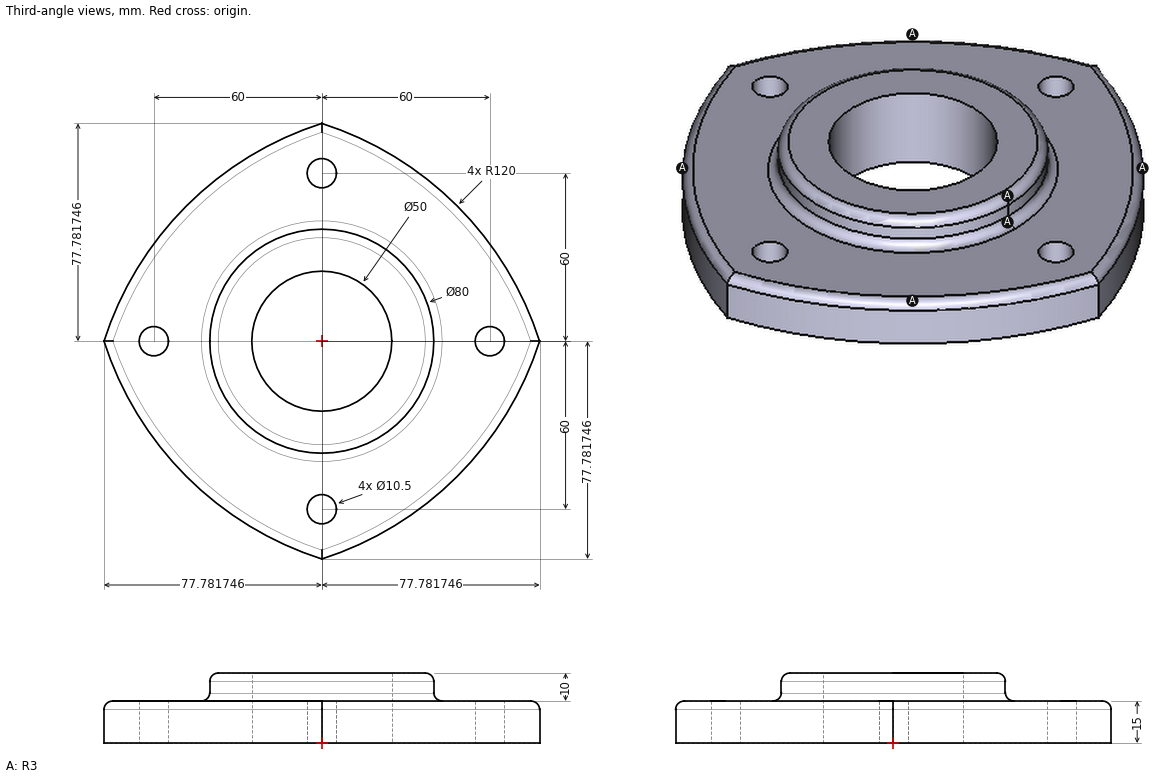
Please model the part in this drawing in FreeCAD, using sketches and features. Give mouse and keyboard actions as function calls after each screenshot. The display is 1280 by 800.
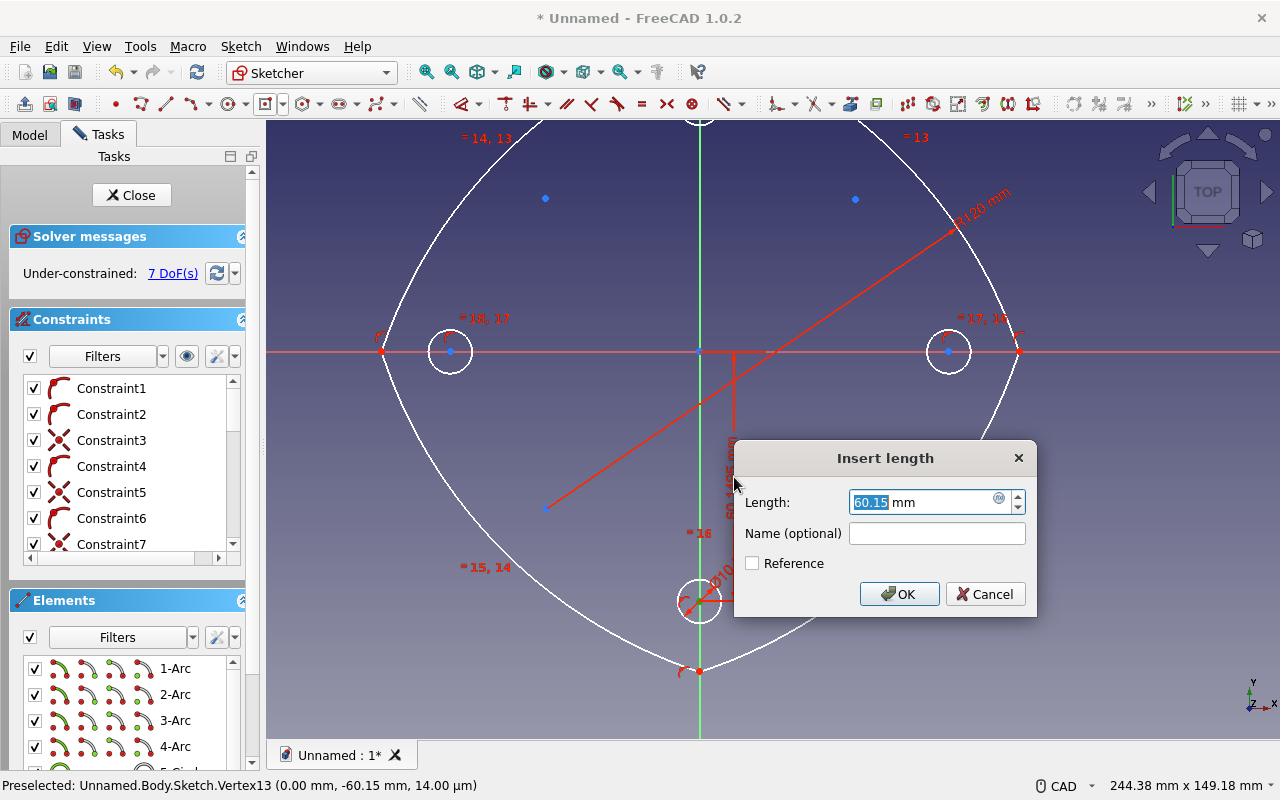
text(60)
key(Return)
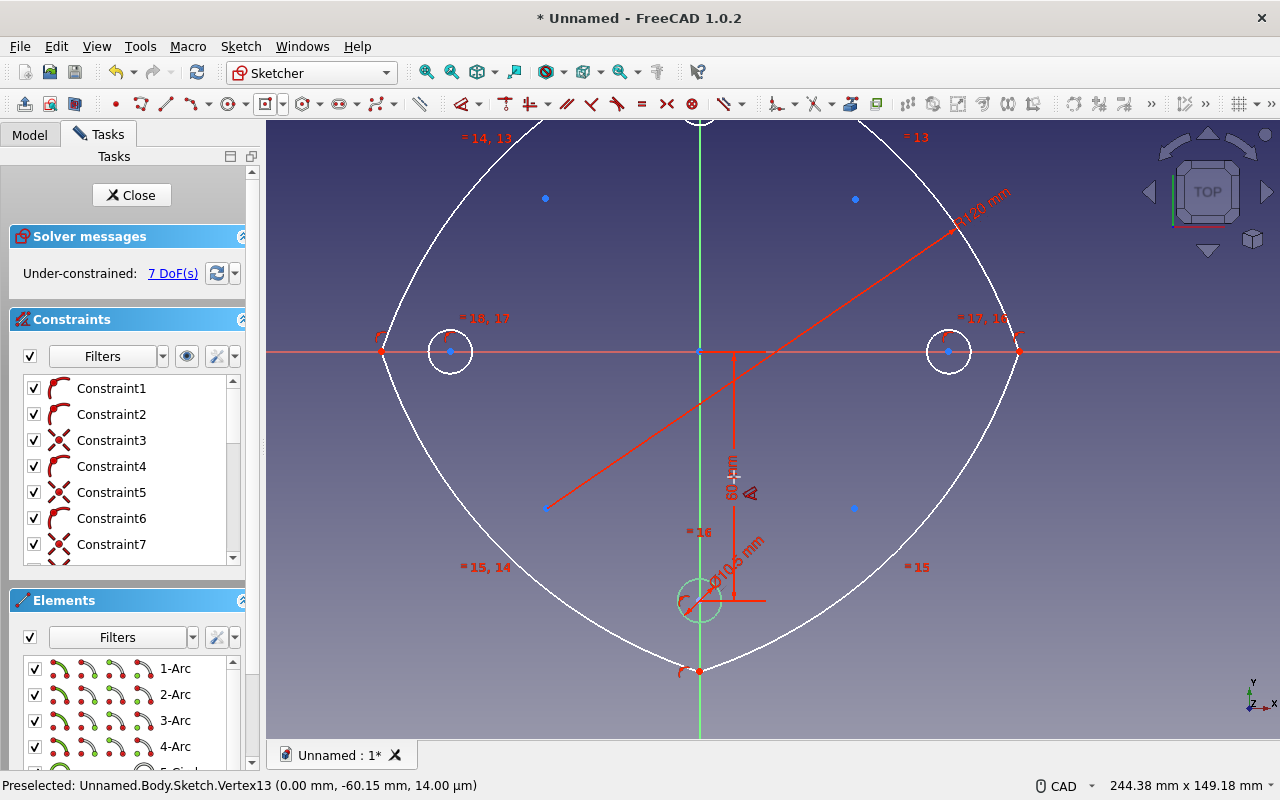
click(949, 352)
click(824, 386)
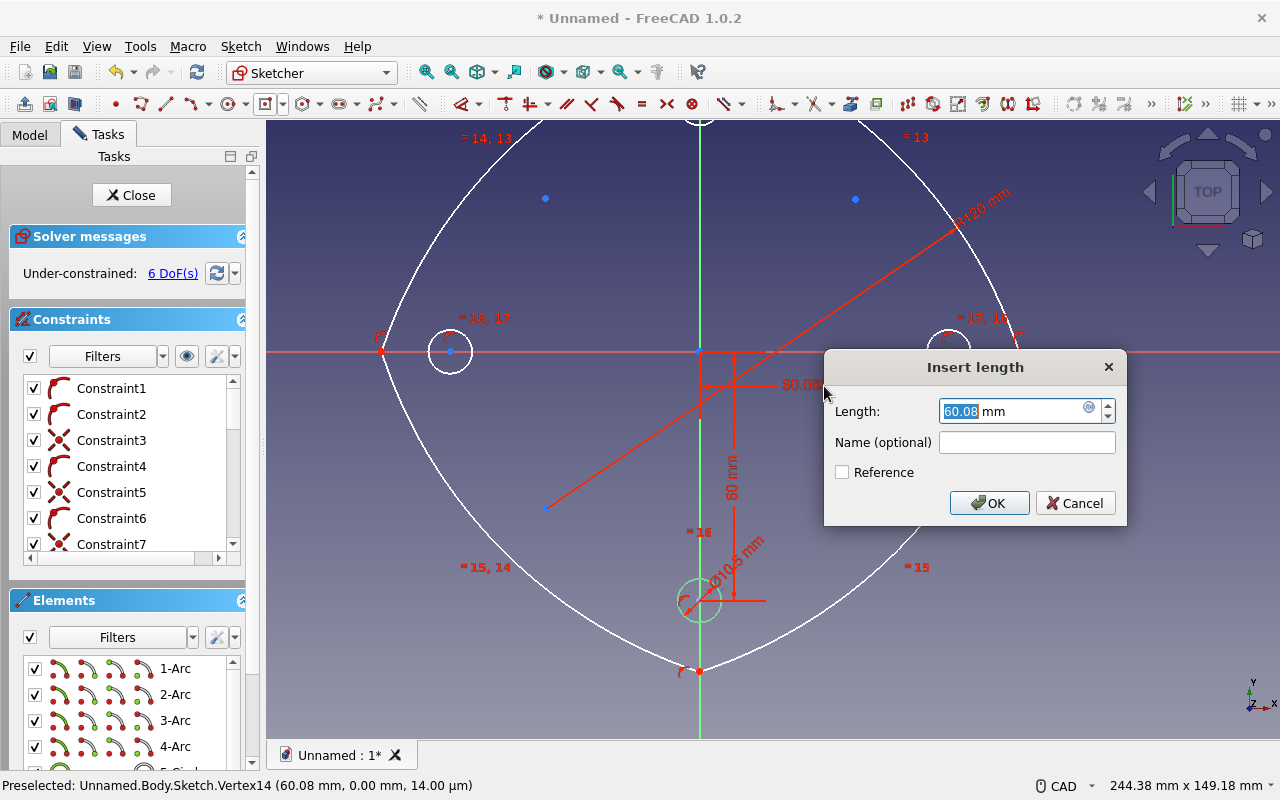
text(60)
key(Return)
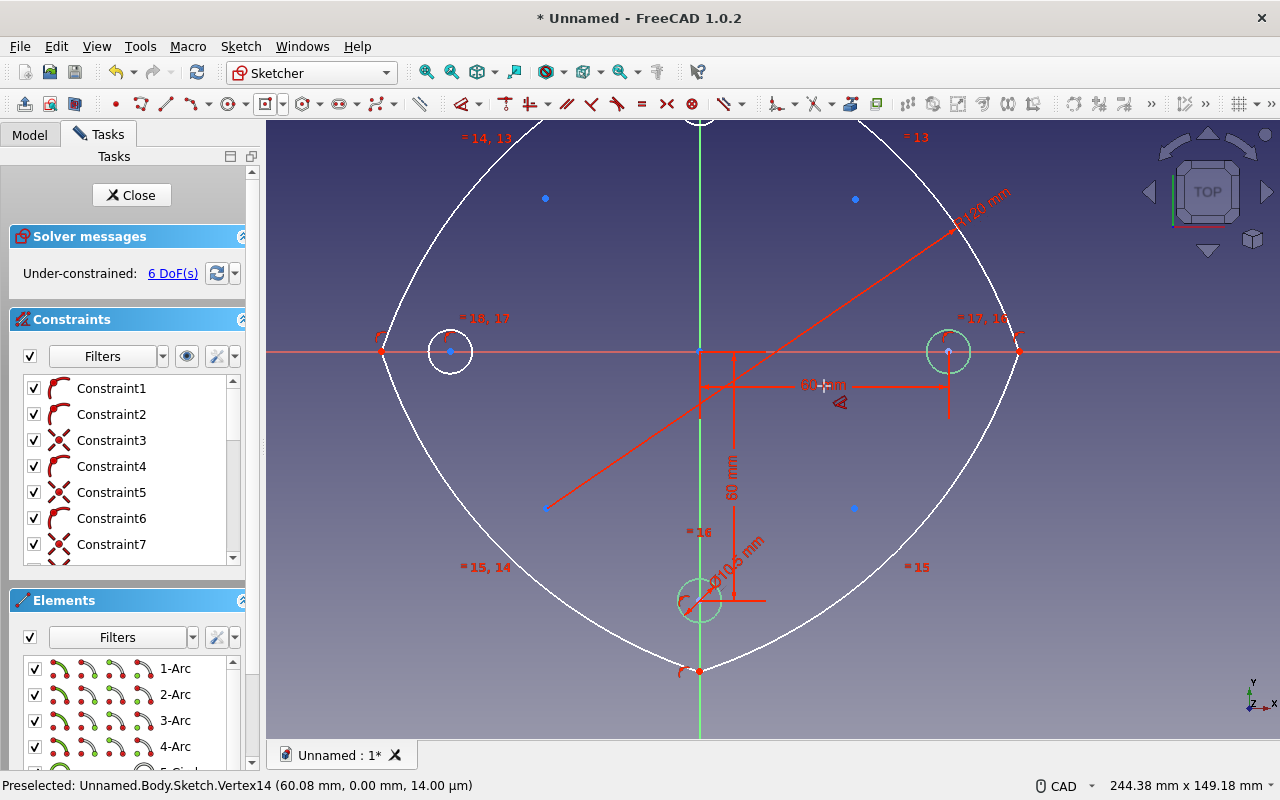
click(450, 352)
click(575, 386)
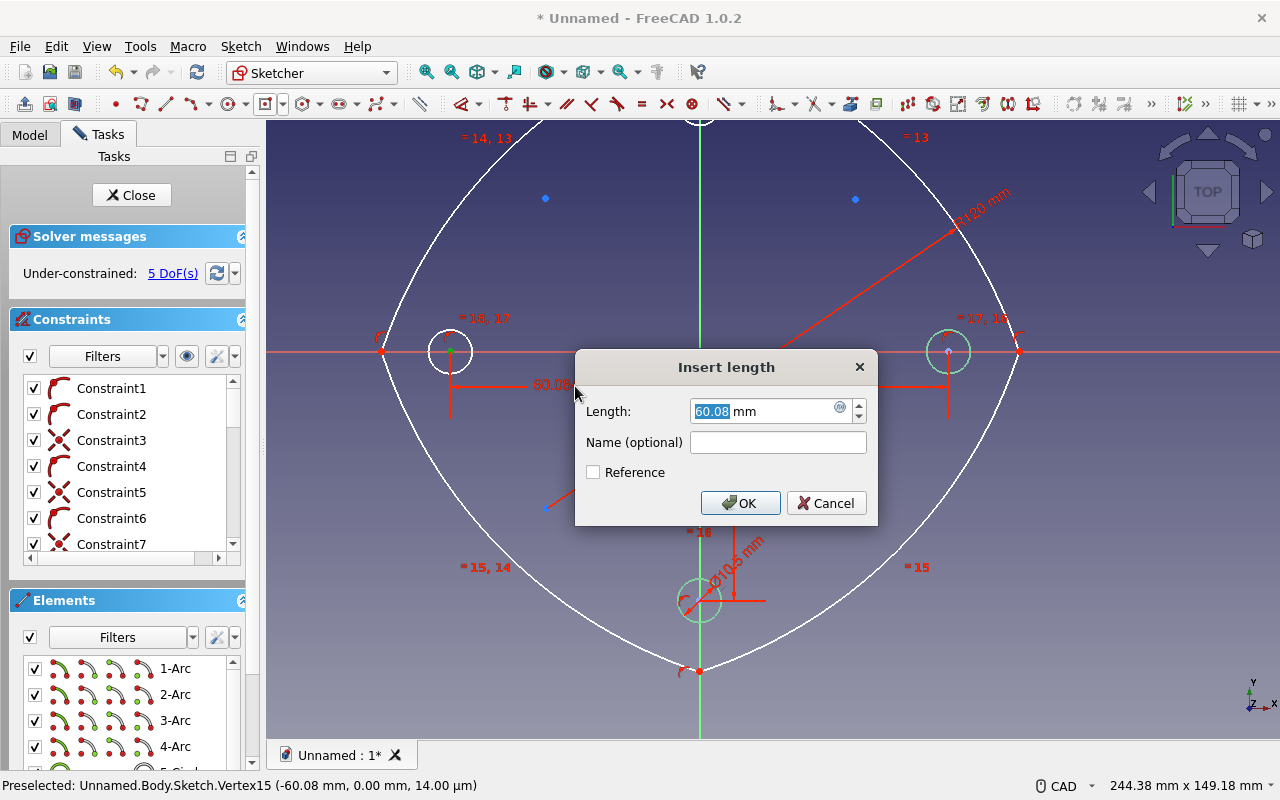
text(60)
key(Return)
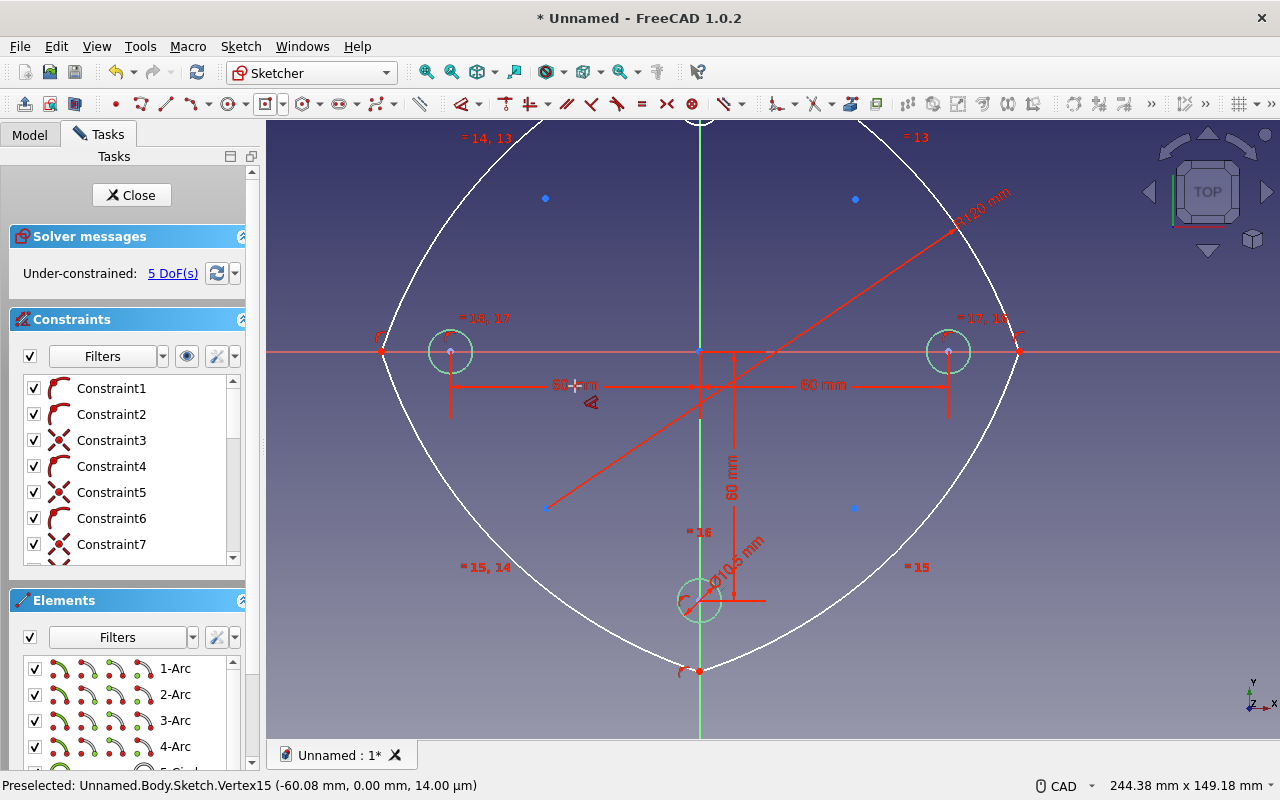
scroll(715, 587, down, 2)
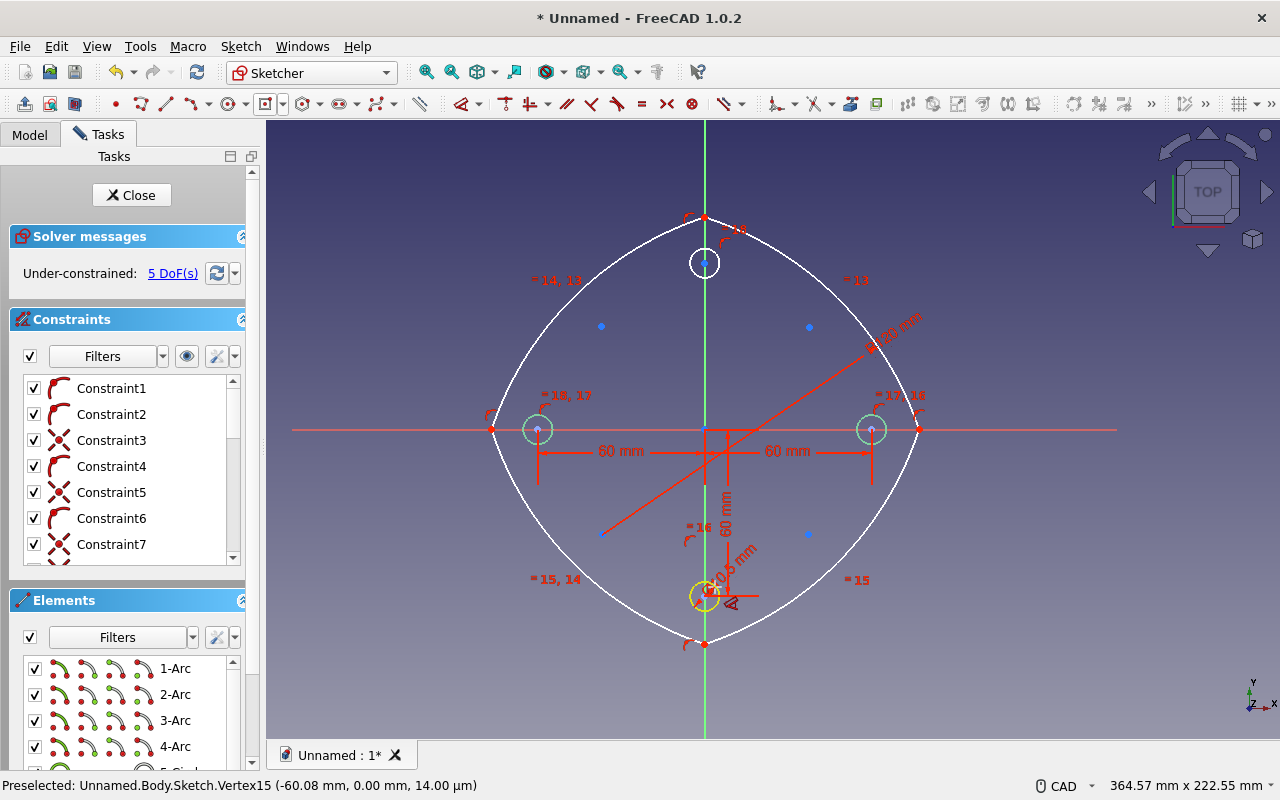
click(705, 263)
click(739, 346)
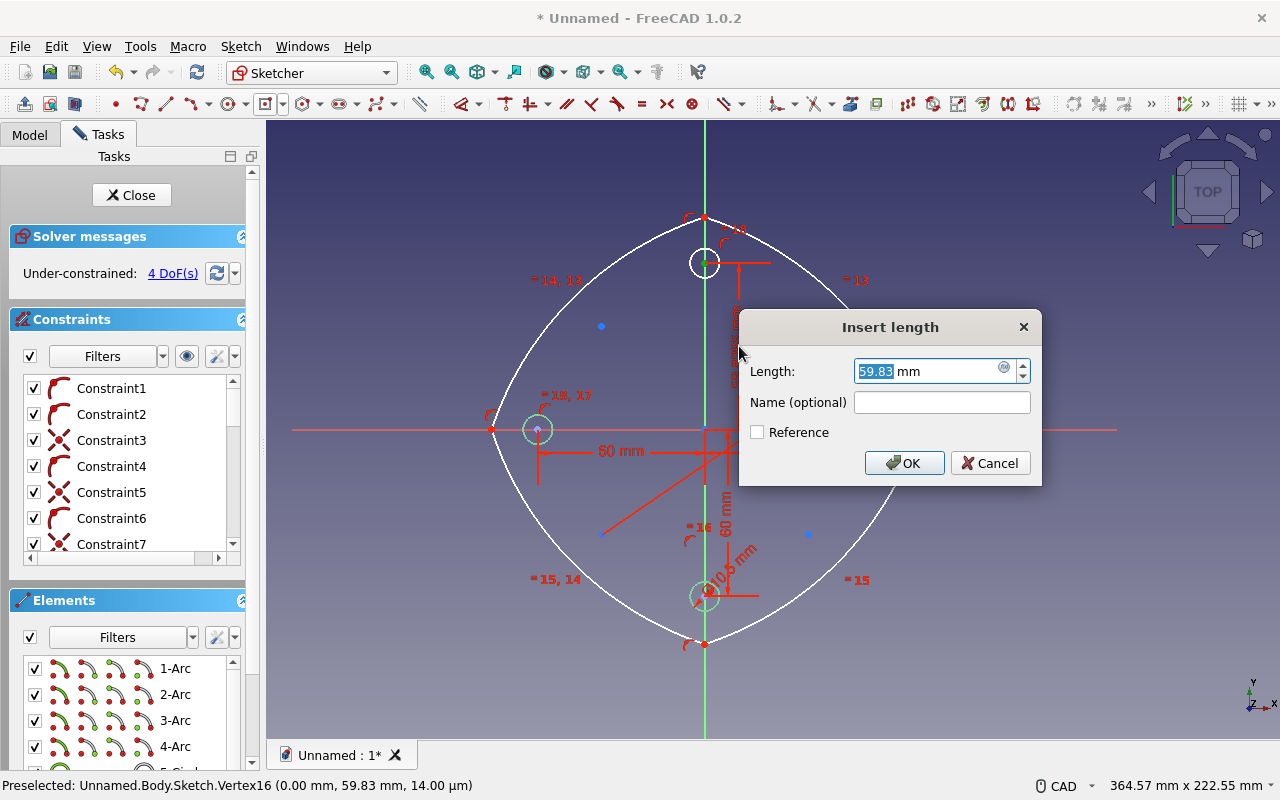
text(60)
key(Return)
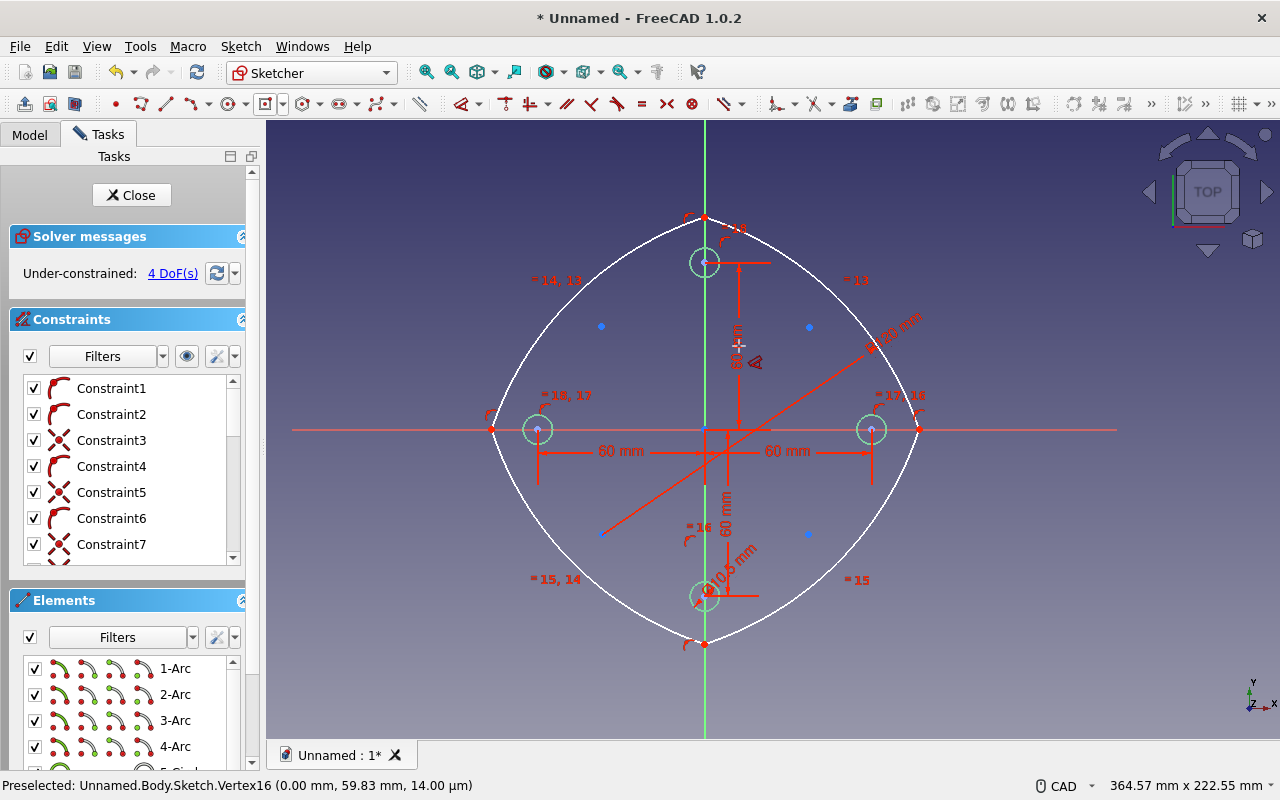
click(919, 430)
click(861, 464)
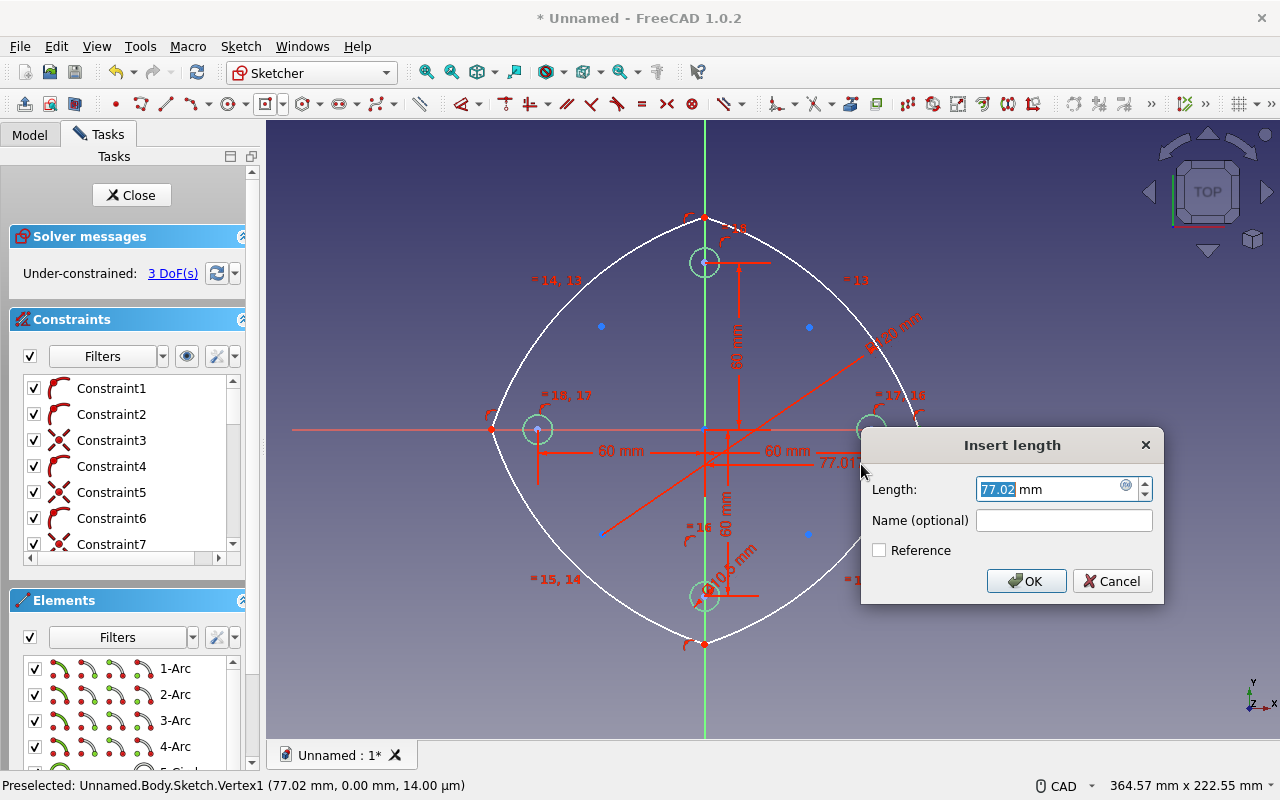
text(77.781746)
key(Return)